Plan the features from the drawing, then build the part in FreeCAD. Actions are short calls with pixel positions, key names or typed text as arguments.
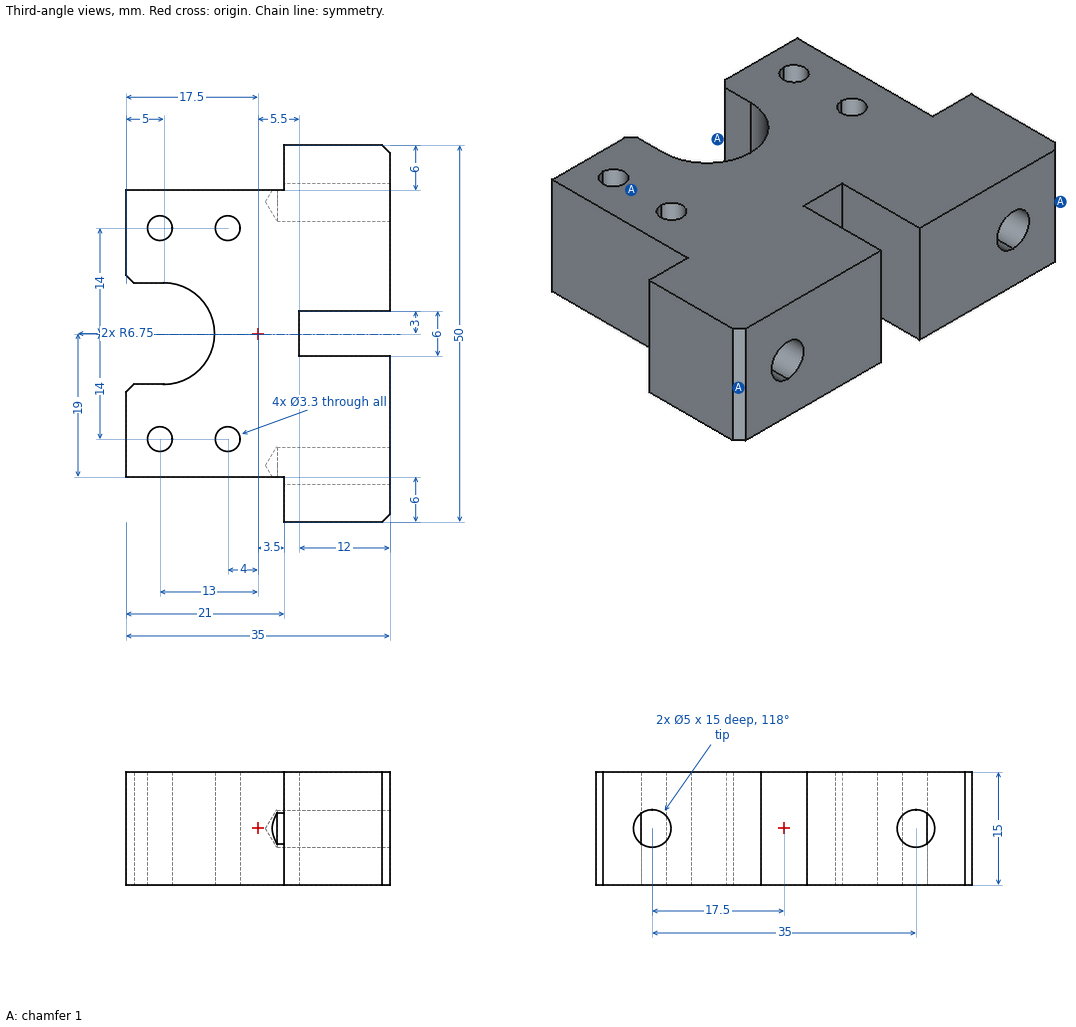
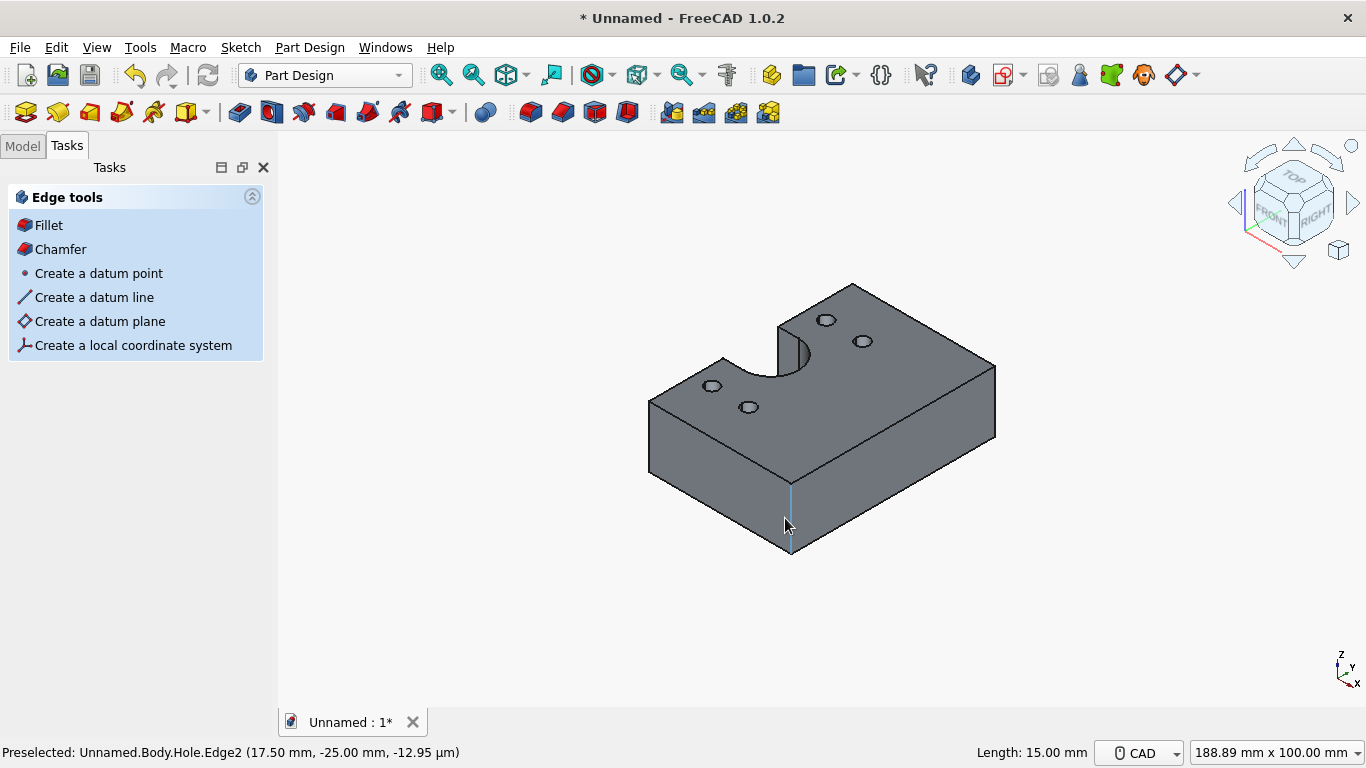
key(2)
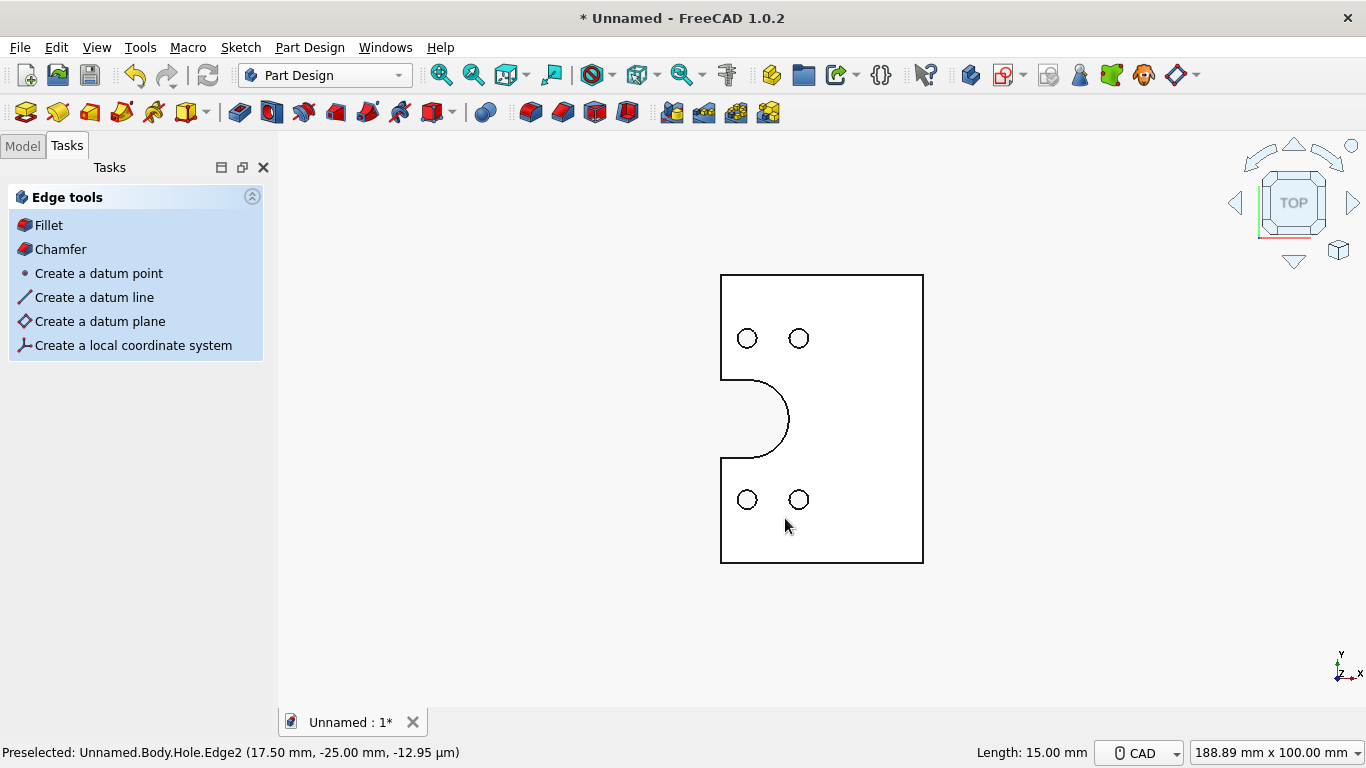
key(1)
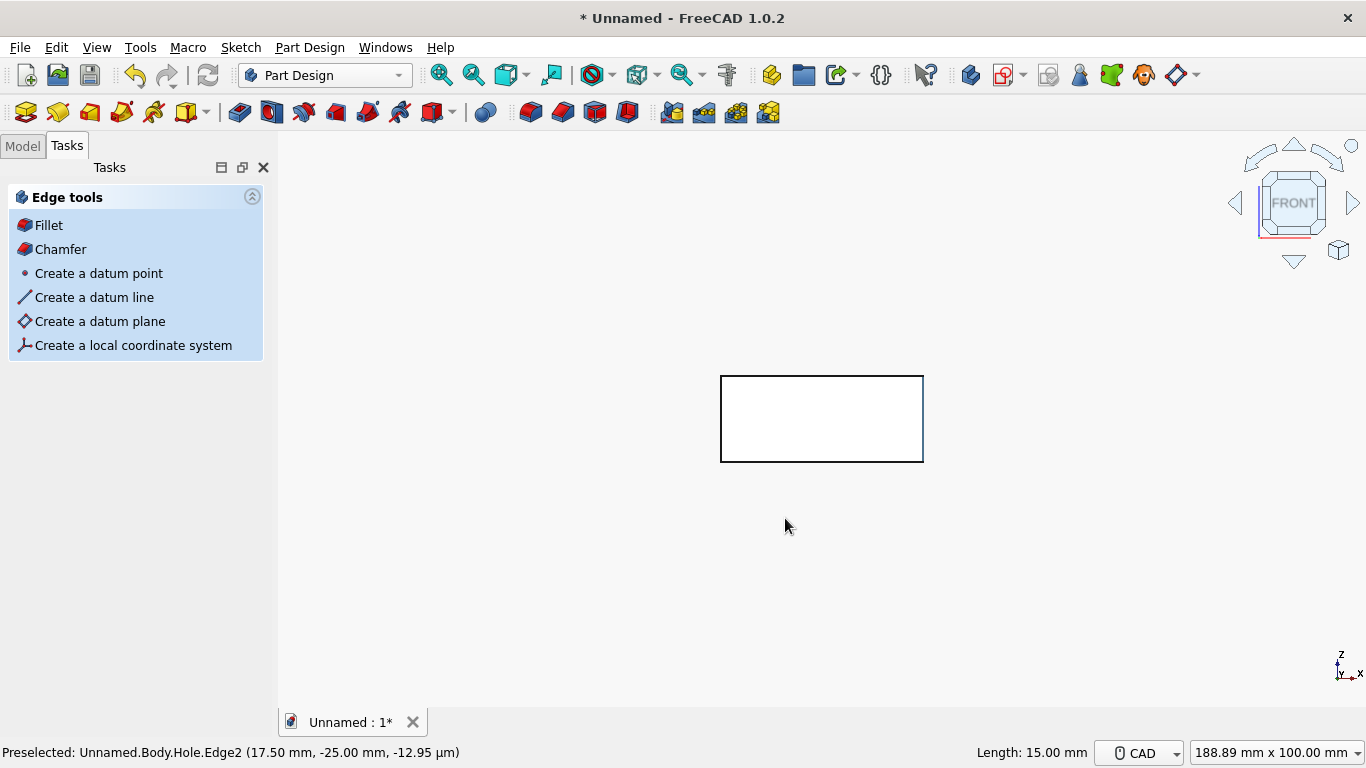
click(442, 76)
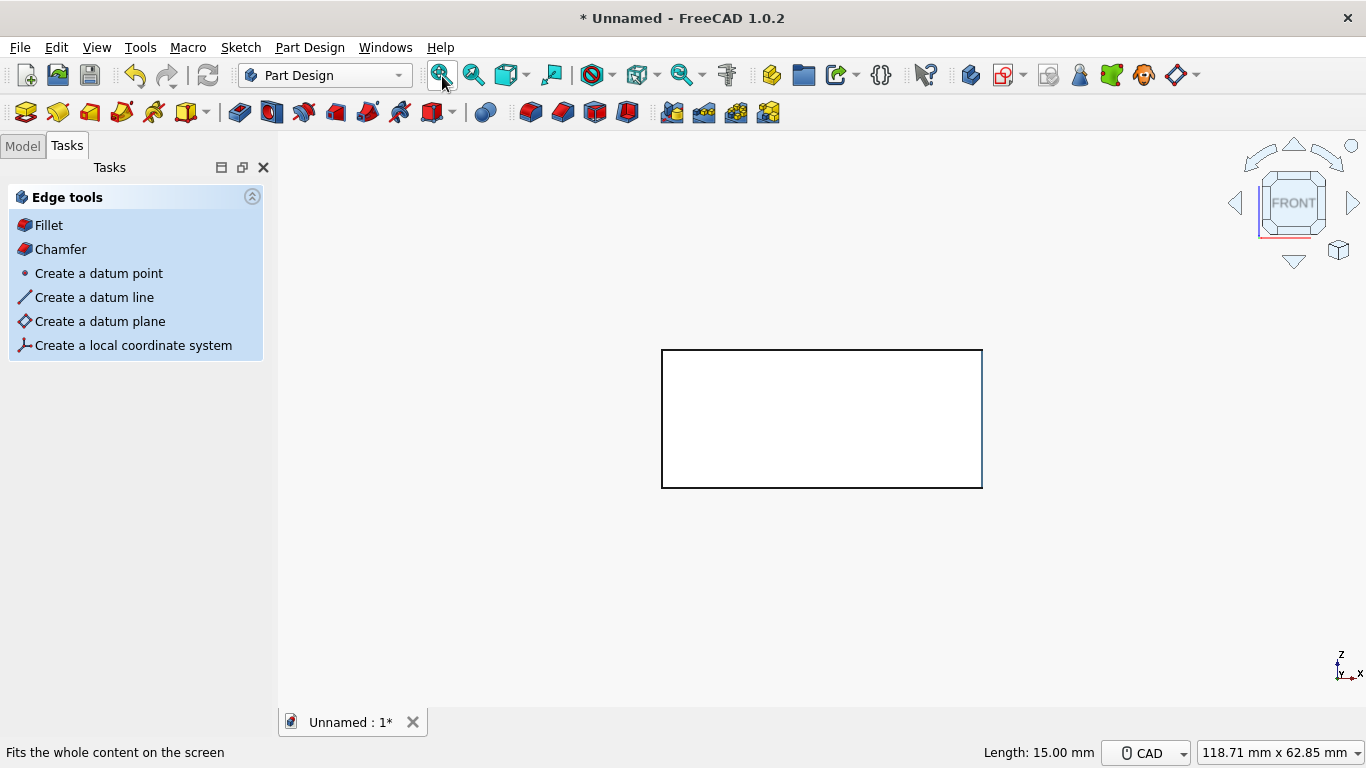
key(3)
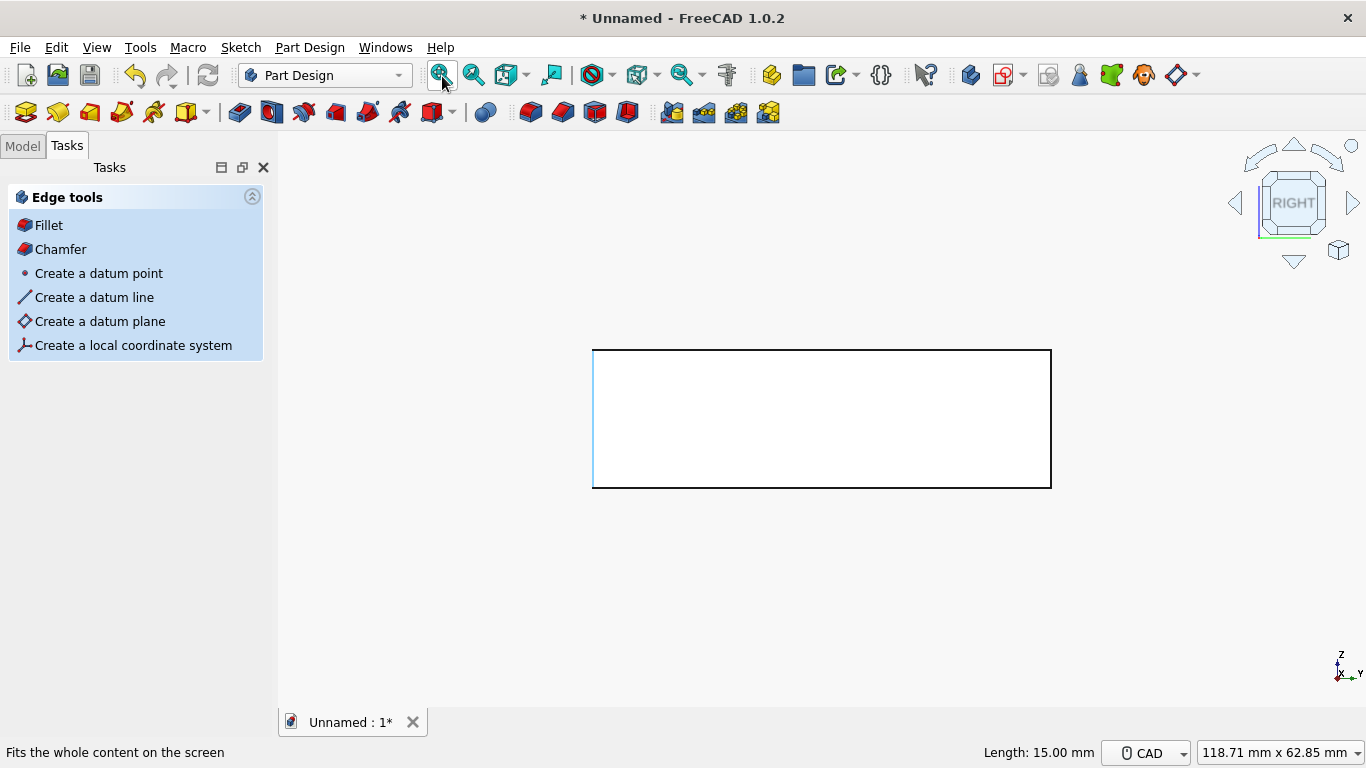
click(442, 76)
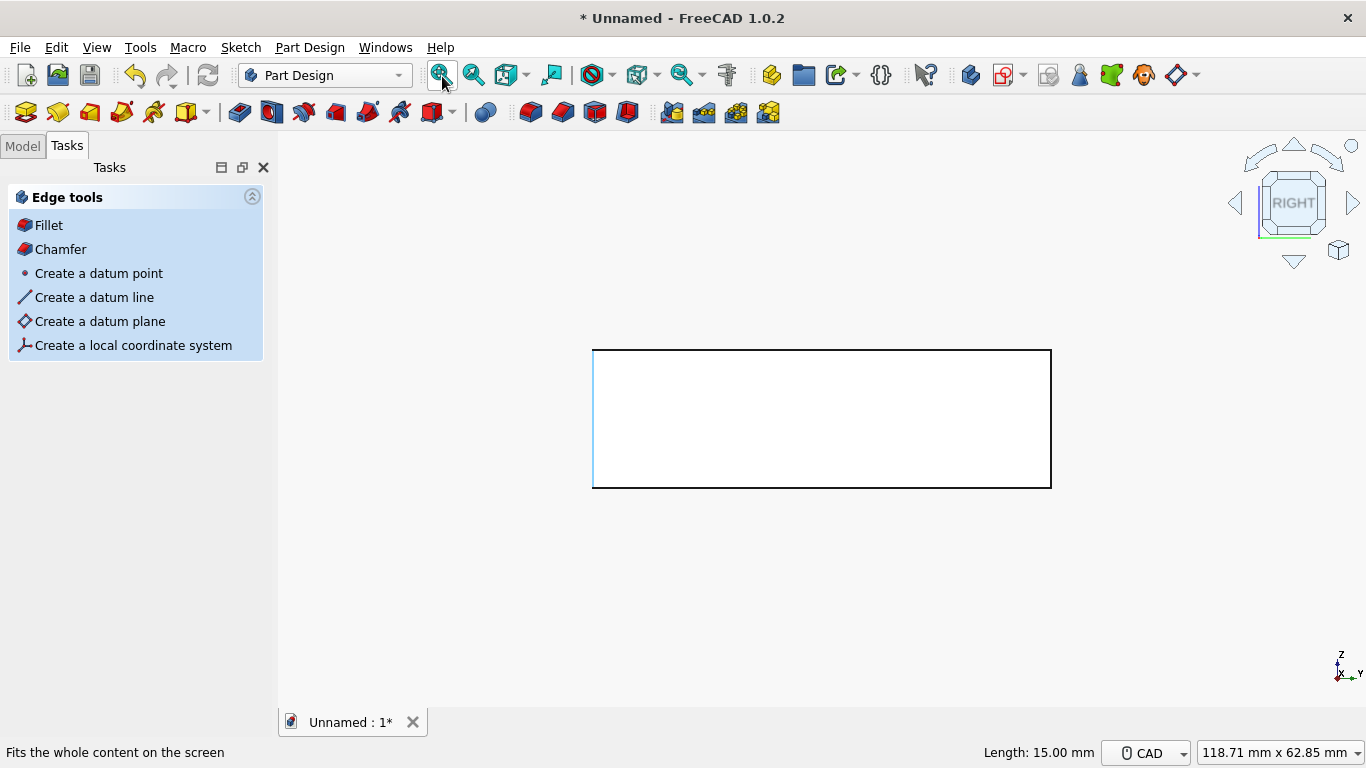
click(1051, 418, ctrl)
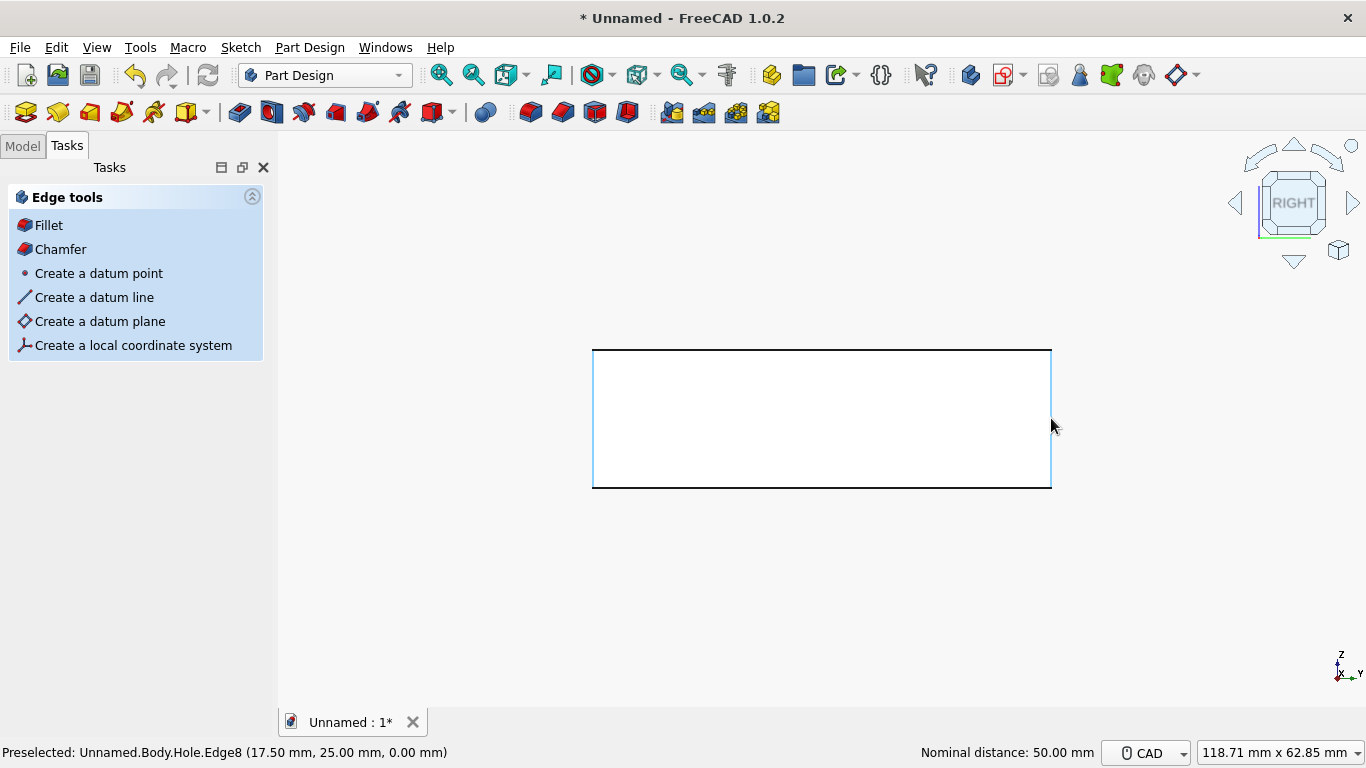
key(5)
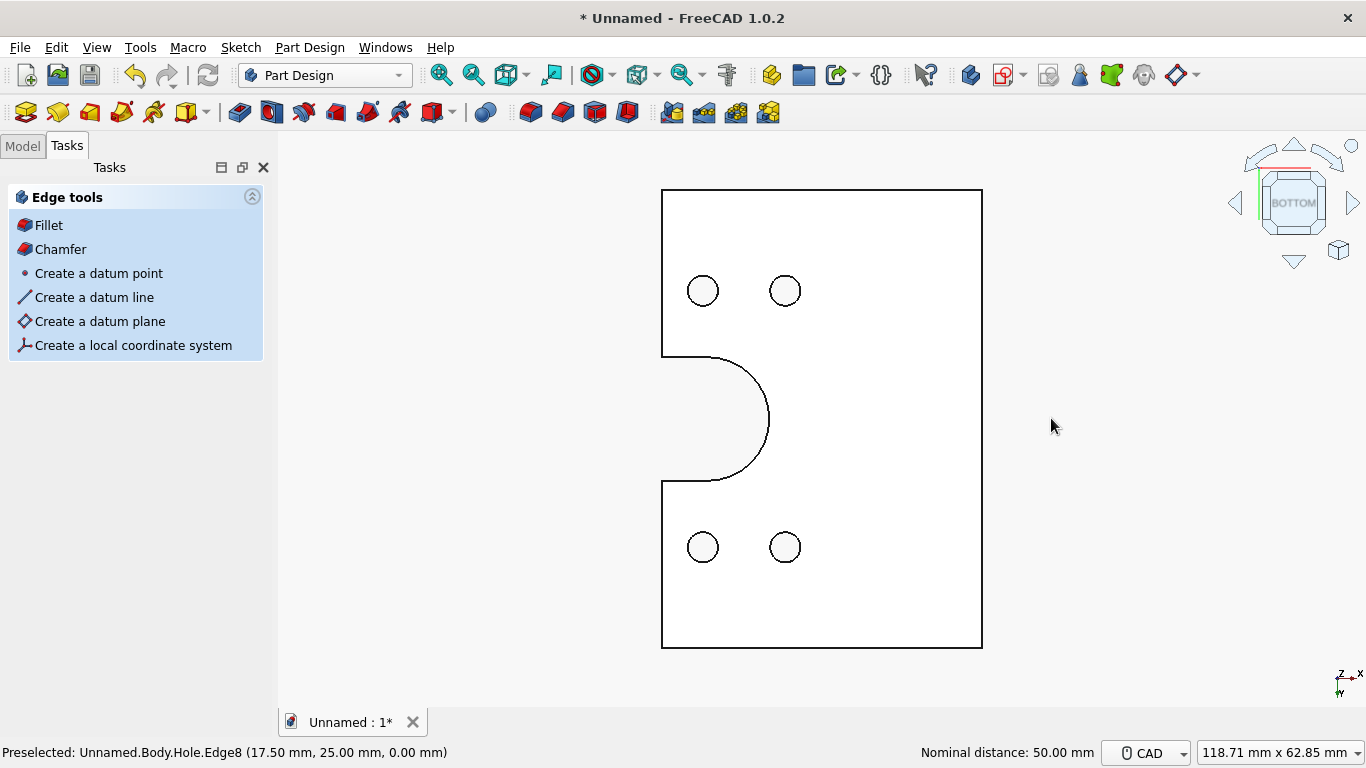
key(4)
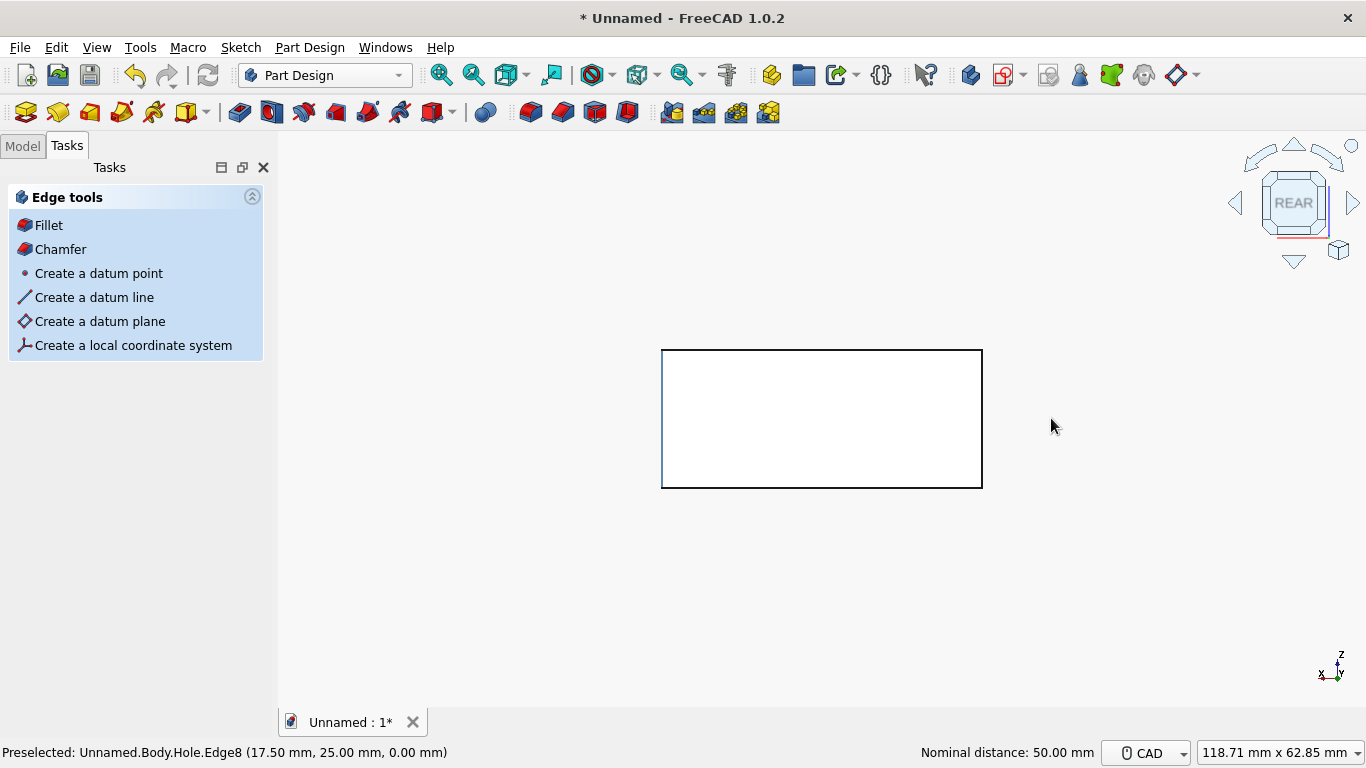
click(442, 76)